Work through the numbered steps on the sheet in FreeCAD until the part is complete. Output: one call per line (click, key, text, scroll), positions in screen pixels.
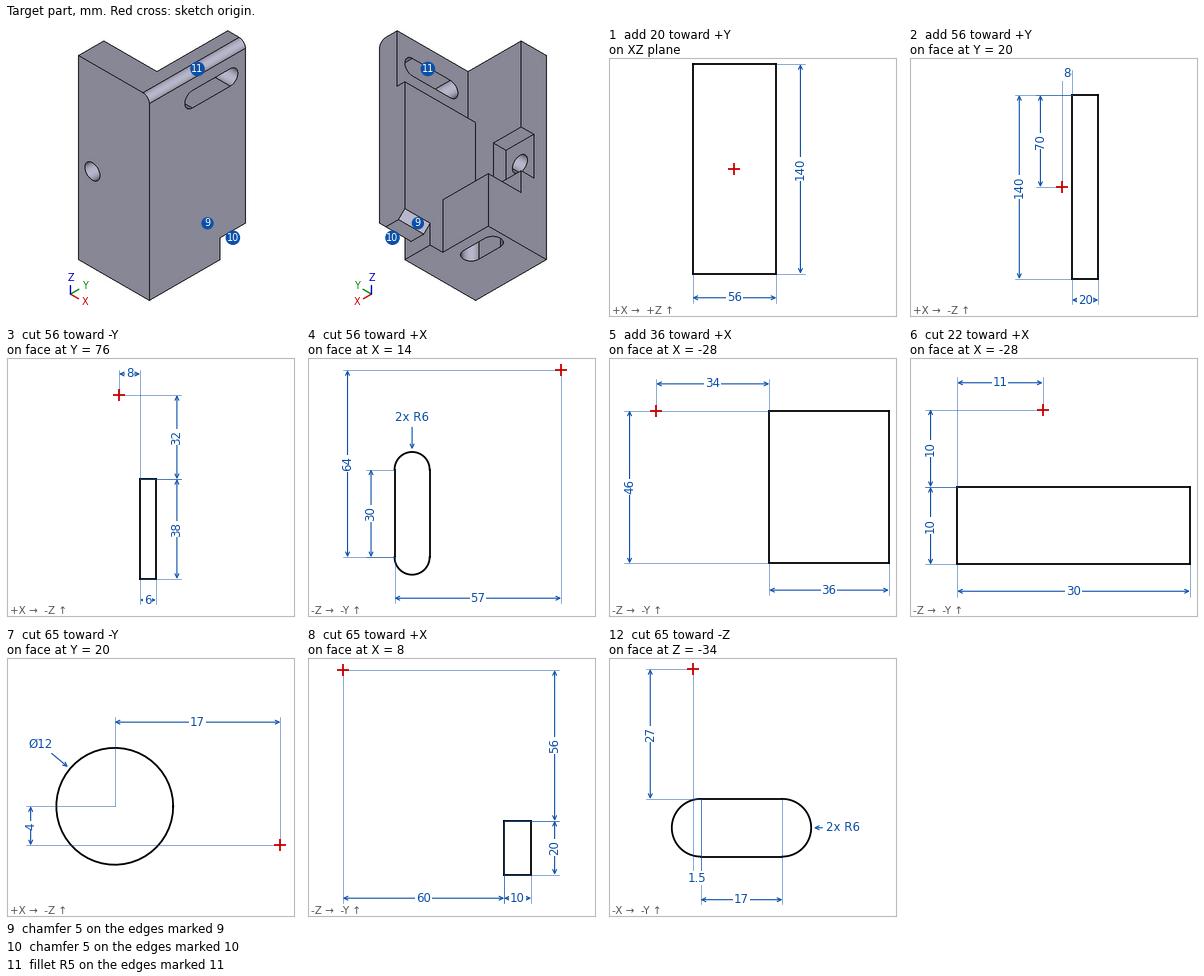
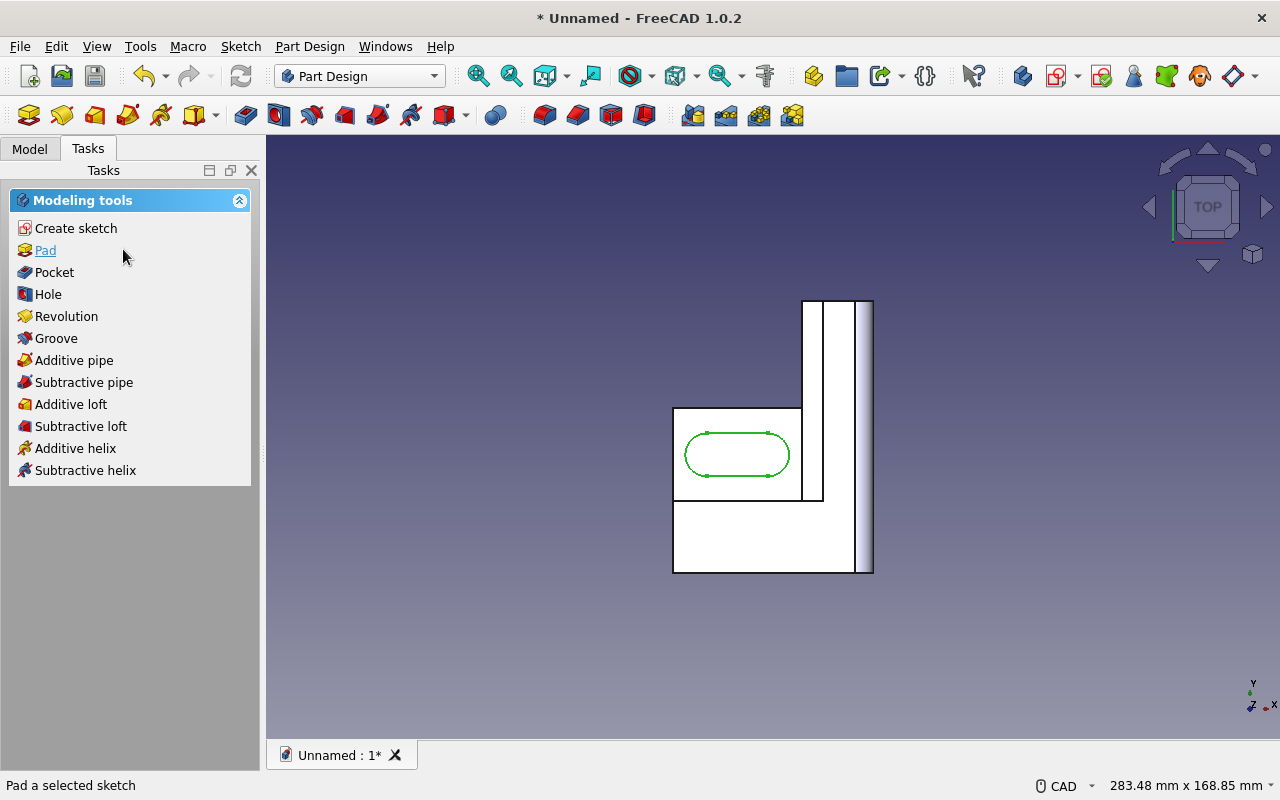
click(246, 116)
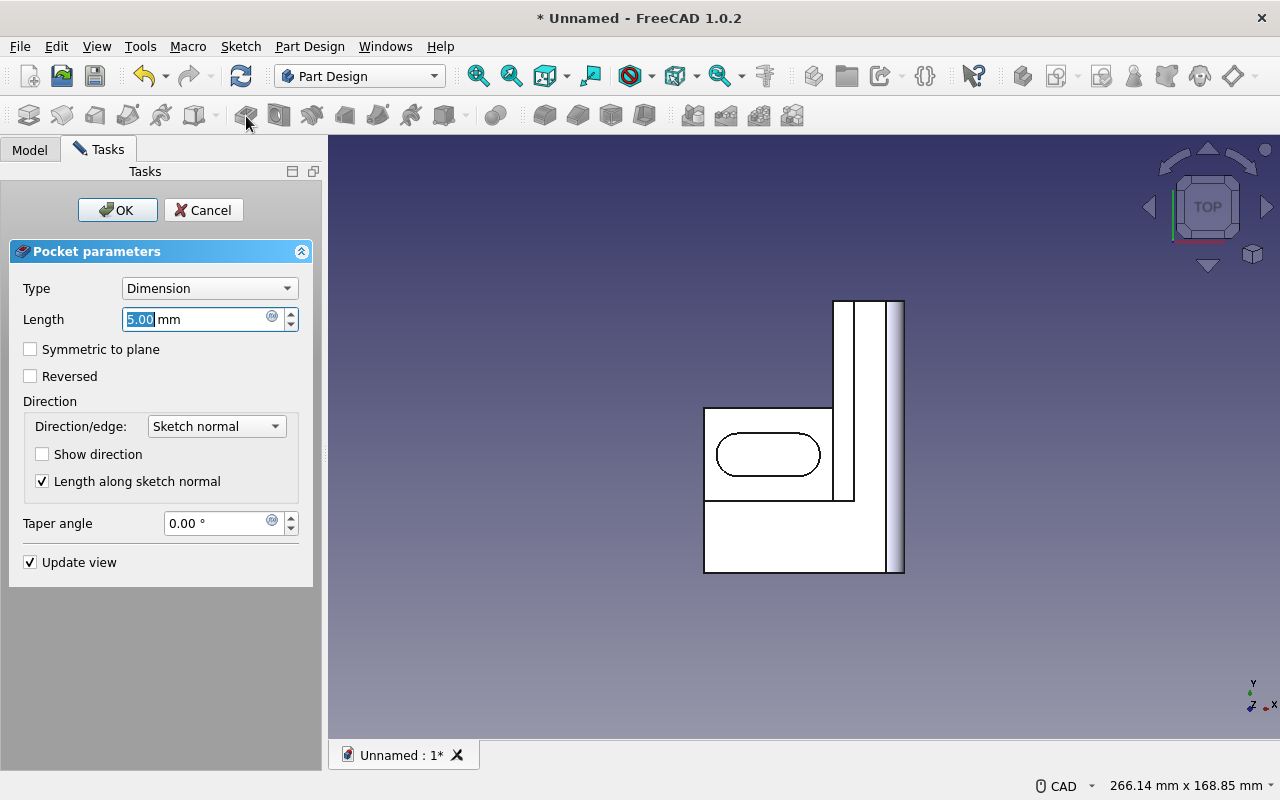
text(65)
key(Tab)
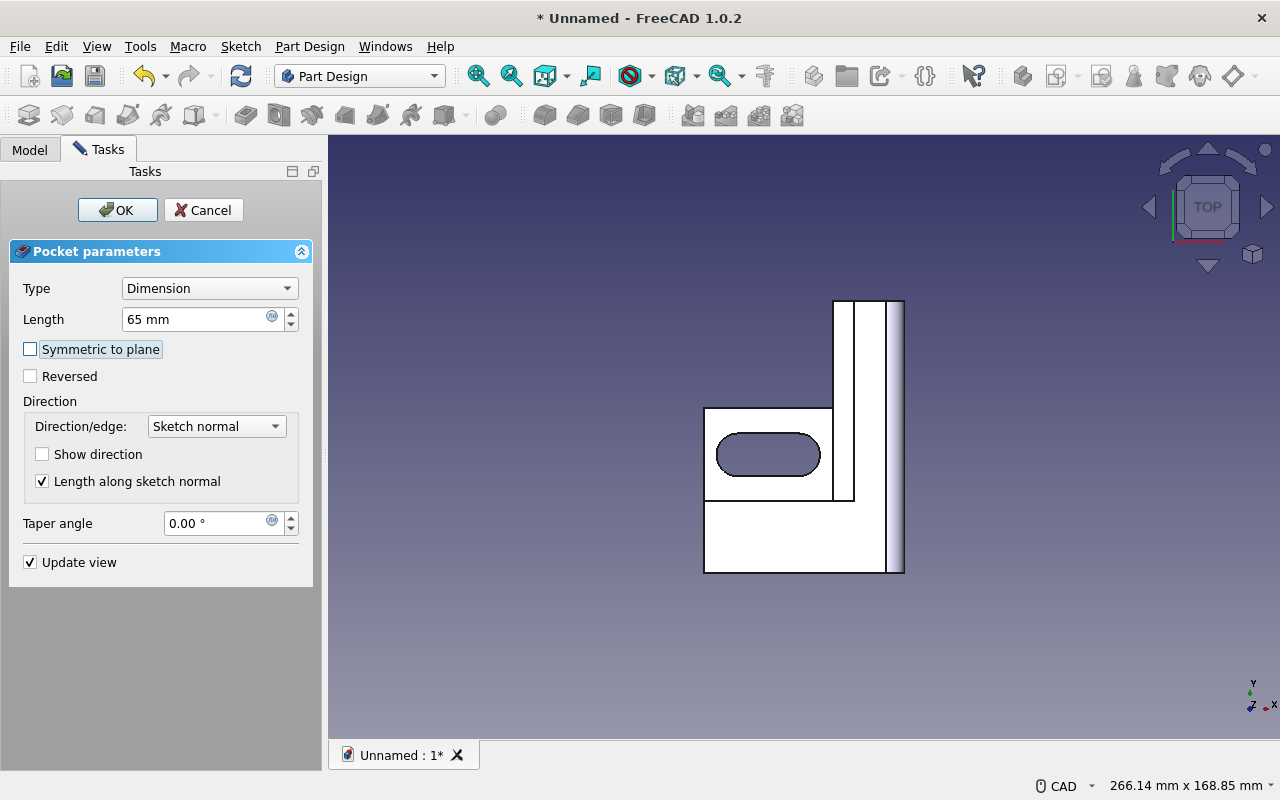
click(118, 210)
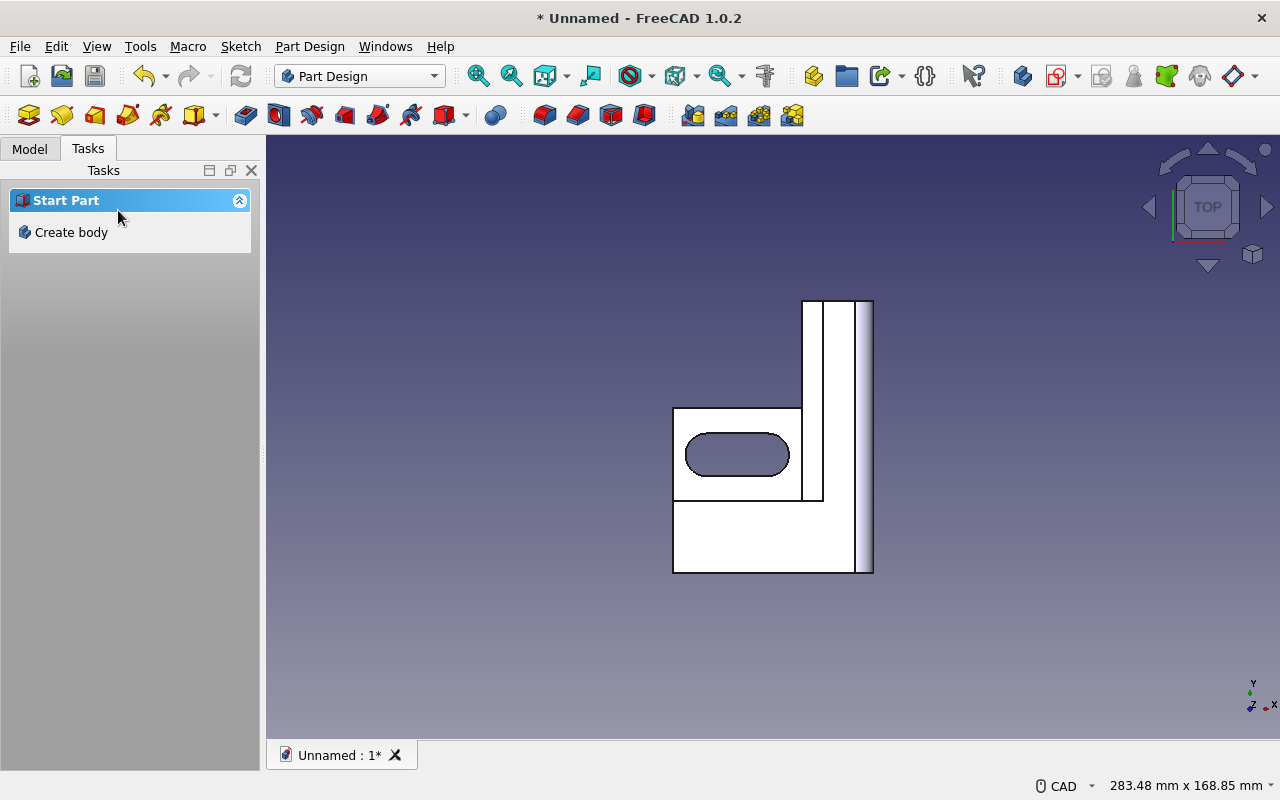
key(0)